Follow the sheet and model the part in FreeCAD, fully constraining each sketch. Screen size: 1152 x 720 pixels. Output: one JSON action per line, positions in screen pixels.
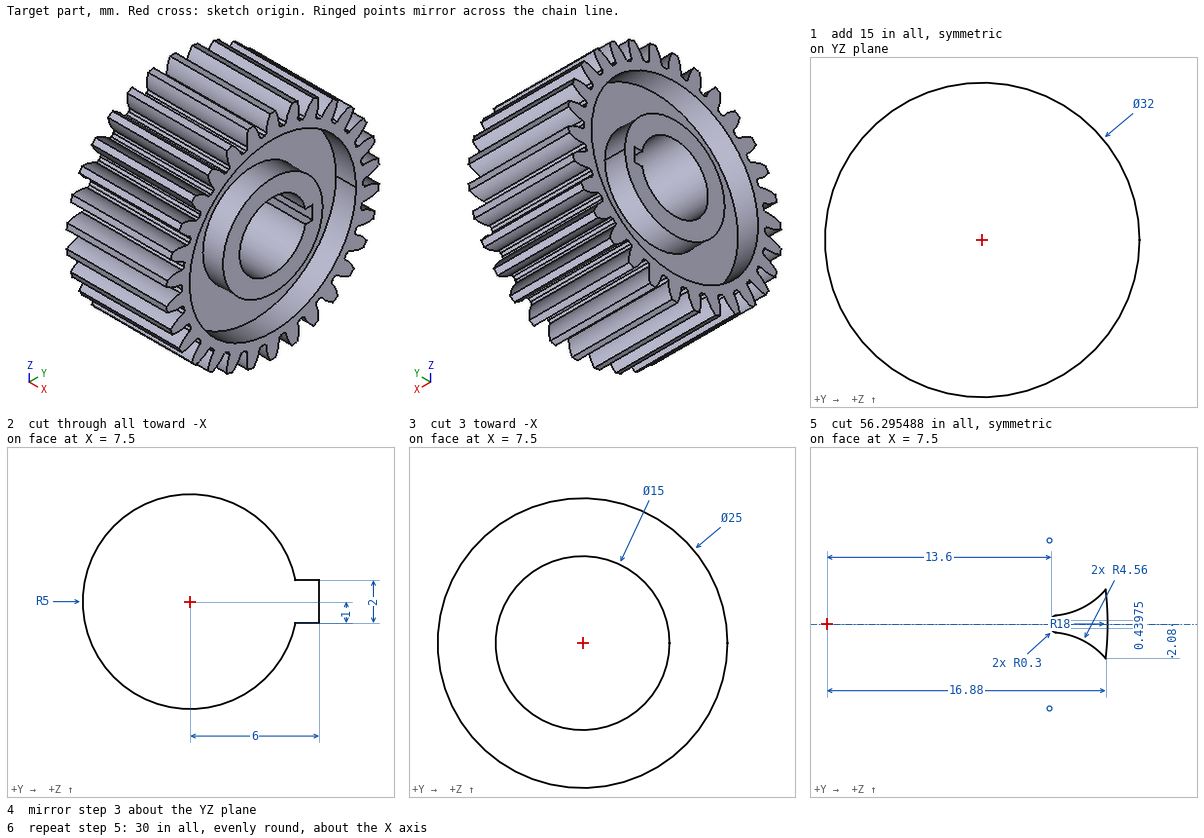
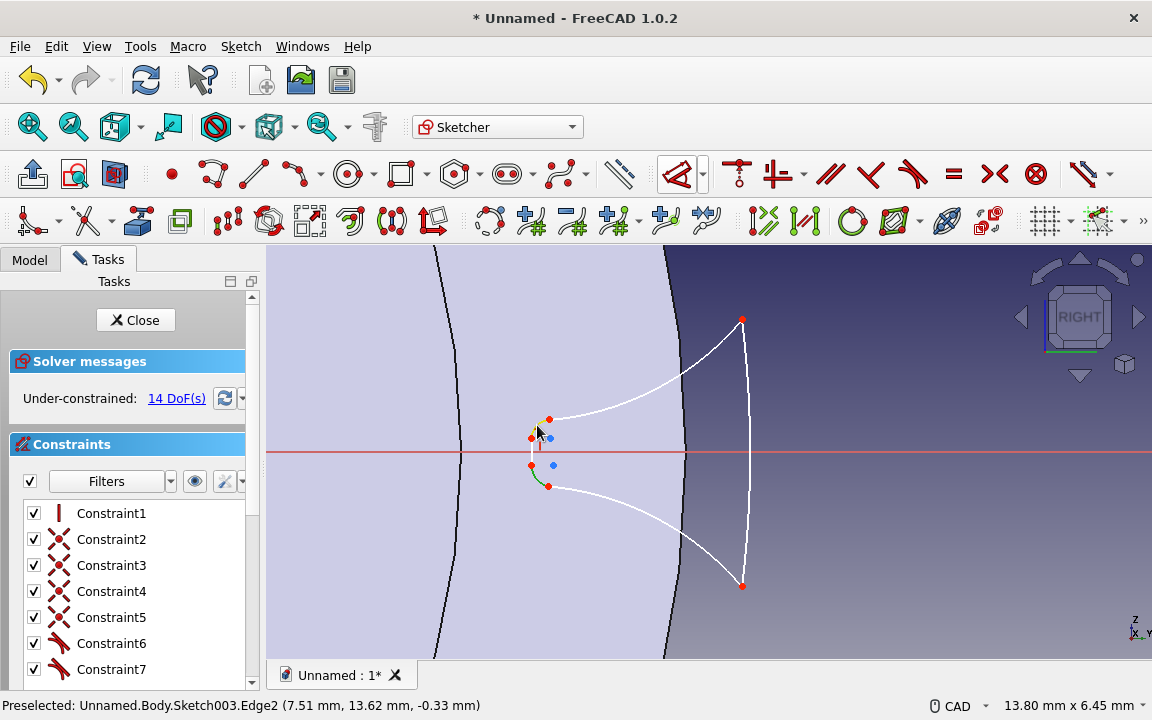
{"action": "left_click", "coordinate": [693, 541]}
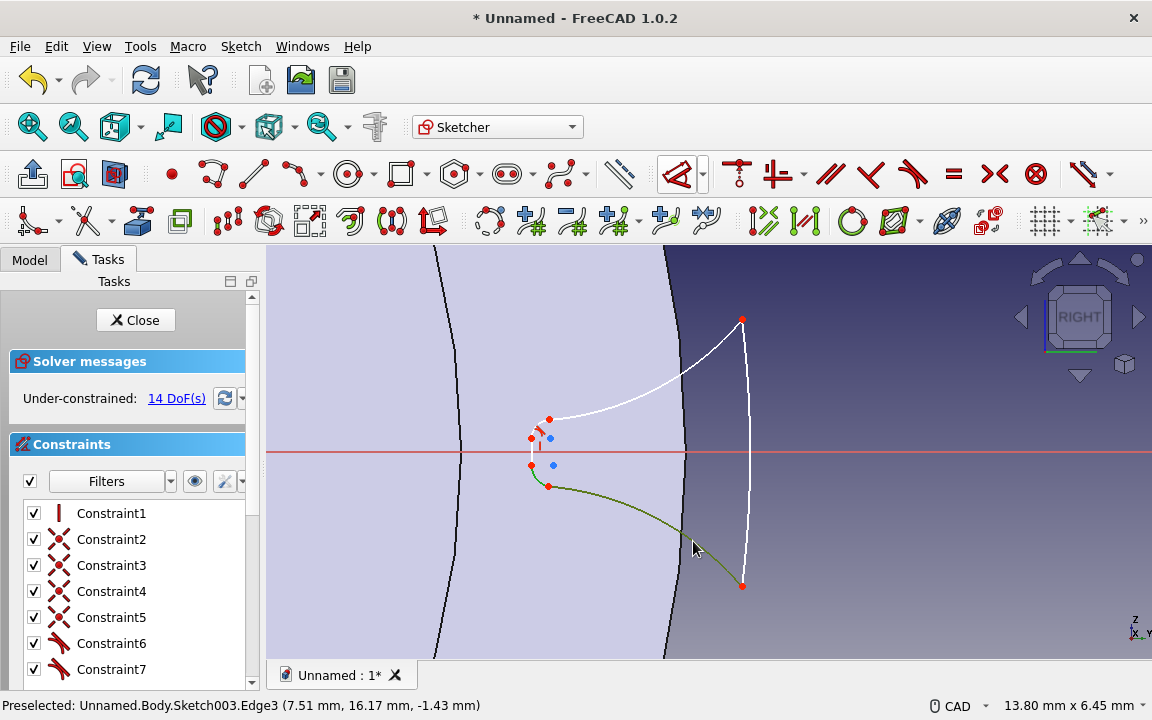
{"action": "left_click", "coordinate": [913, 174]}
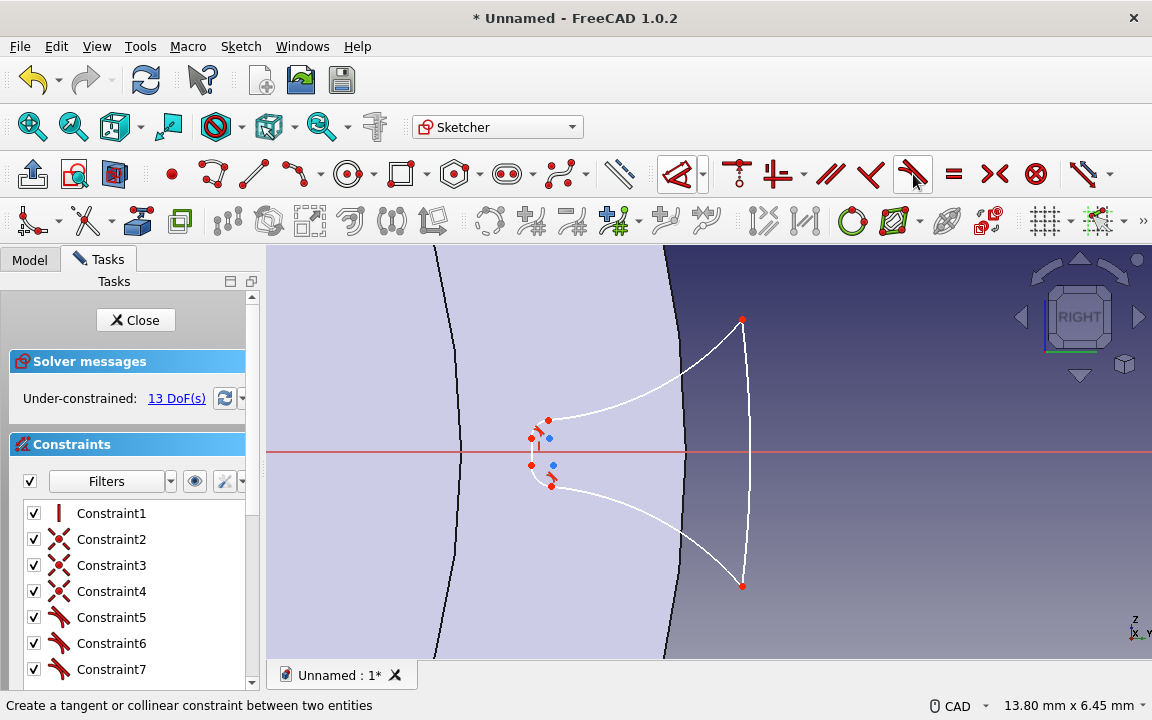
{"action": "left_click", "coordinate": [614, 407]}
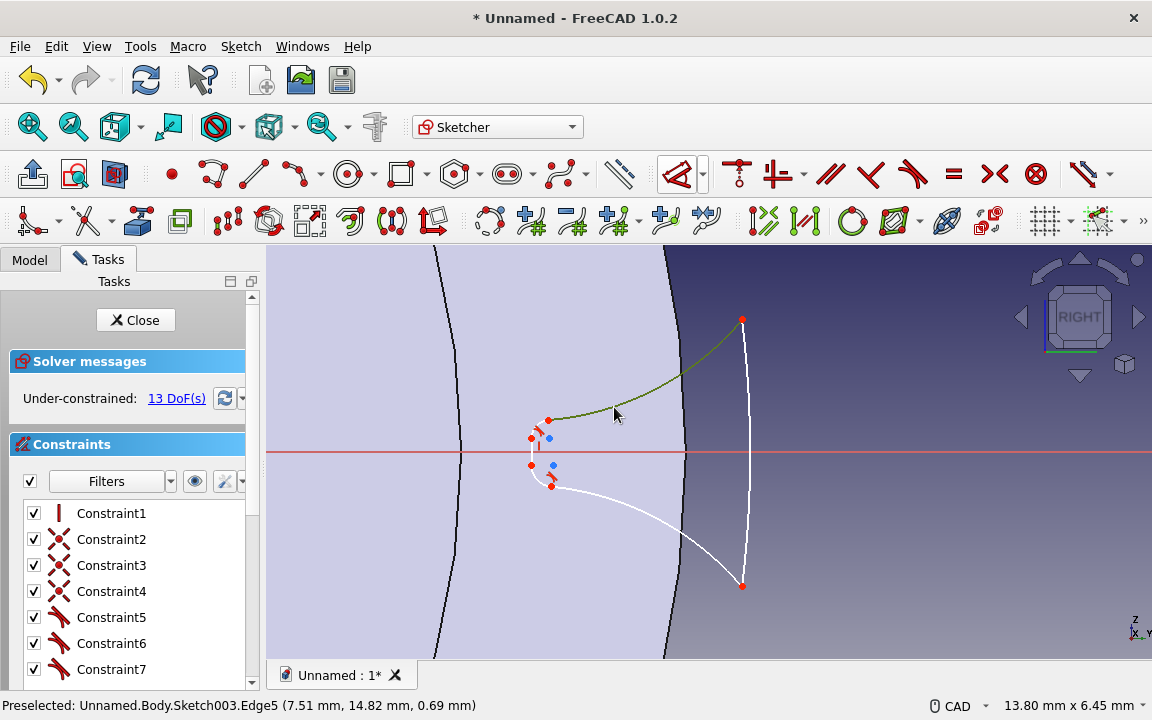
{"action": "left_click", "coordinate": [541, 422]}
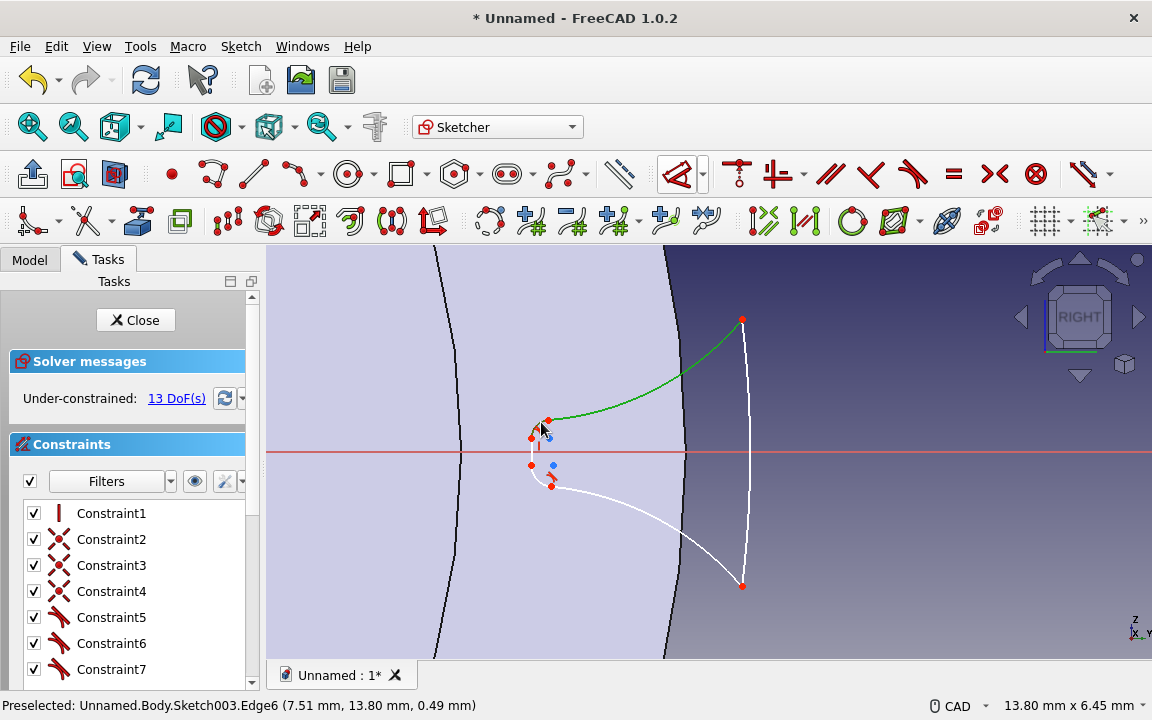
{"action": "key", "text": "t"}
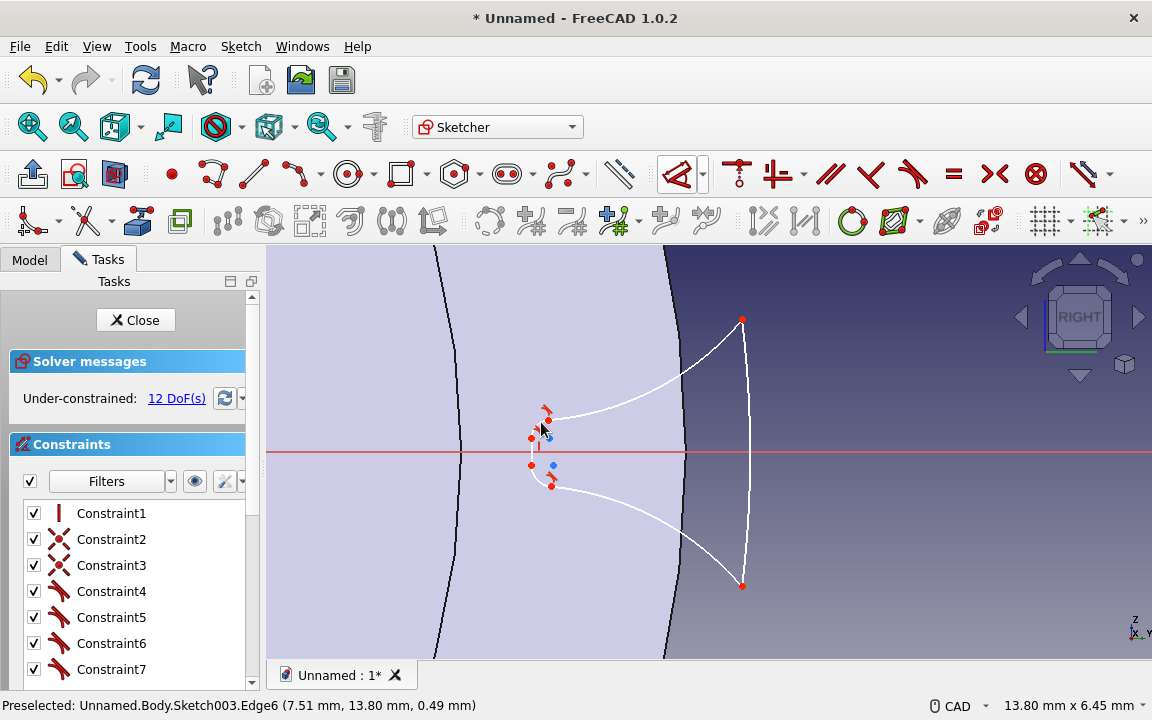
{"action": "left_click", "coordinate": [694, 542]}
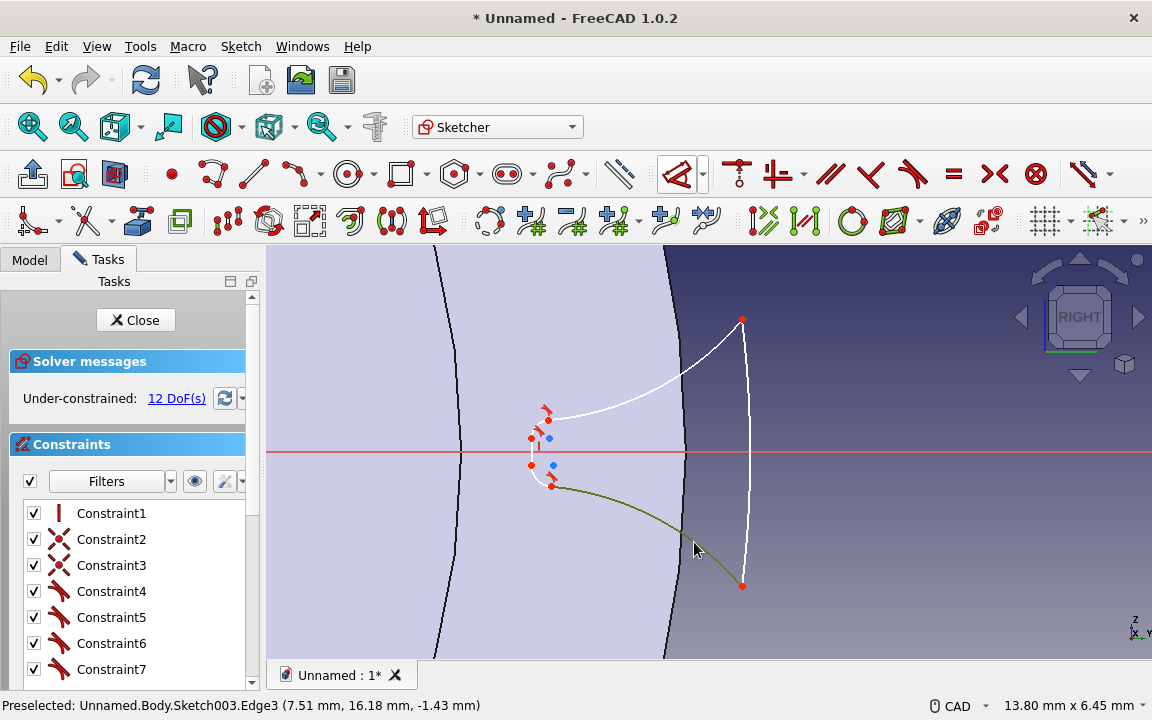
{"action": "left_click", "coordinate": [614, 407]}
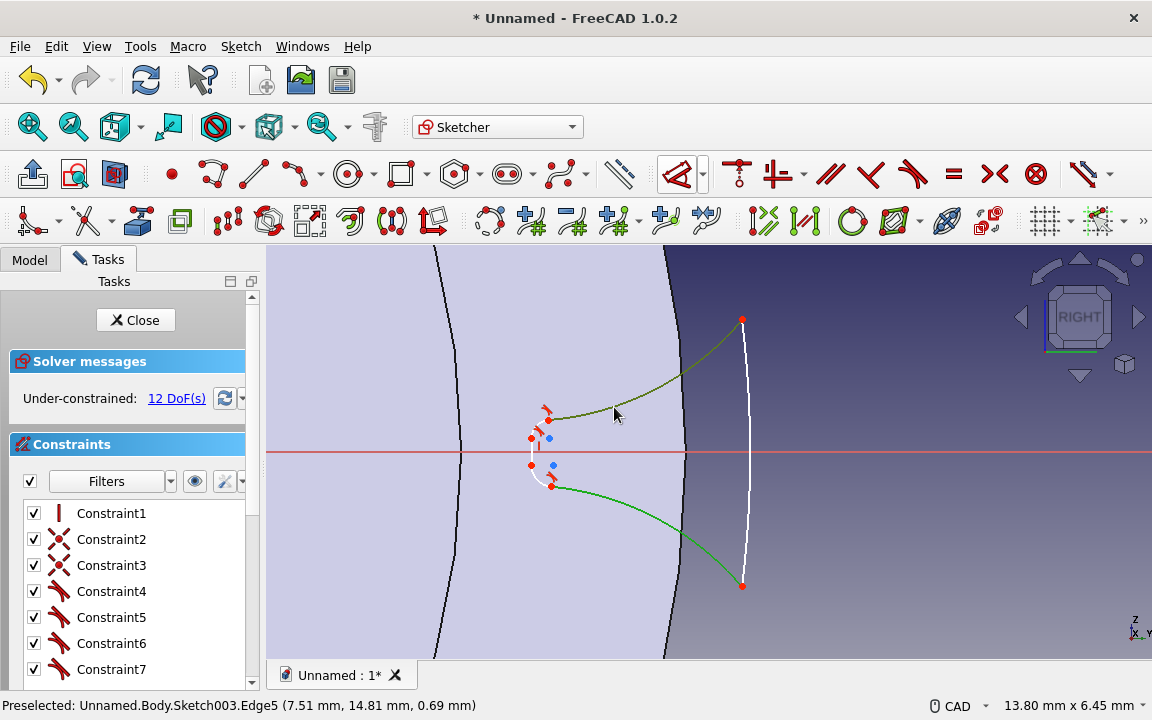
{"action": "key", "text": "e"}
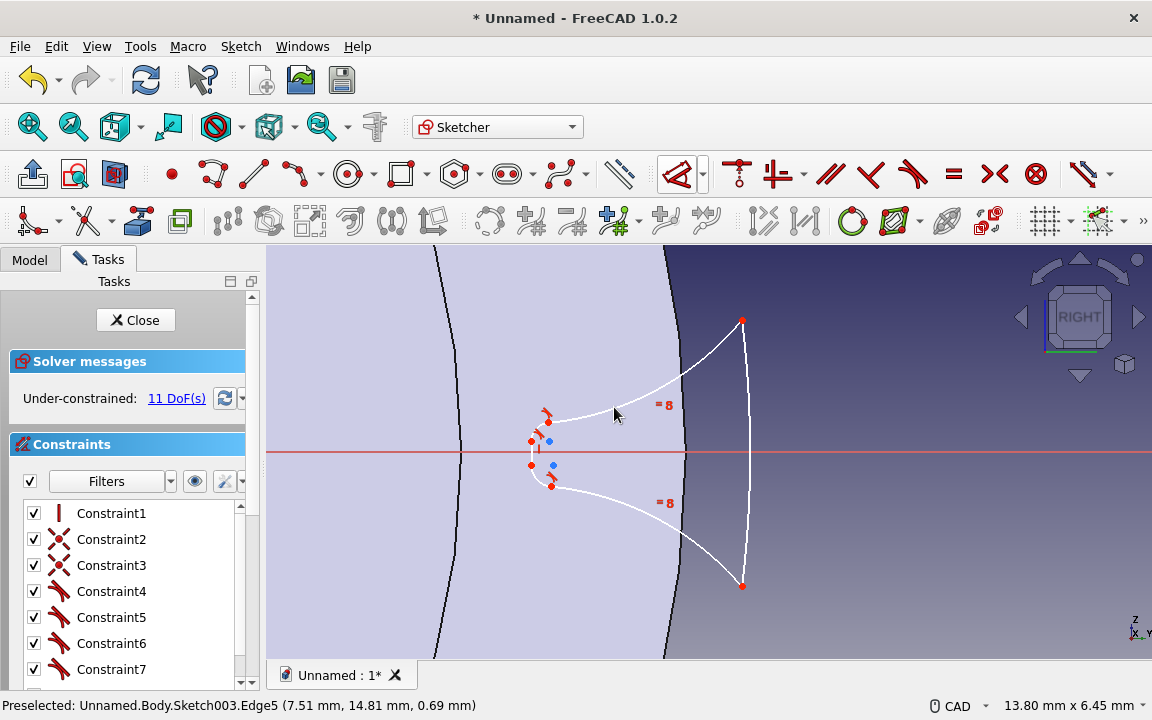
{"action": "scroll", "coordinate": [534, 474], "scroll_direction": "up", "scroll_amount": 2}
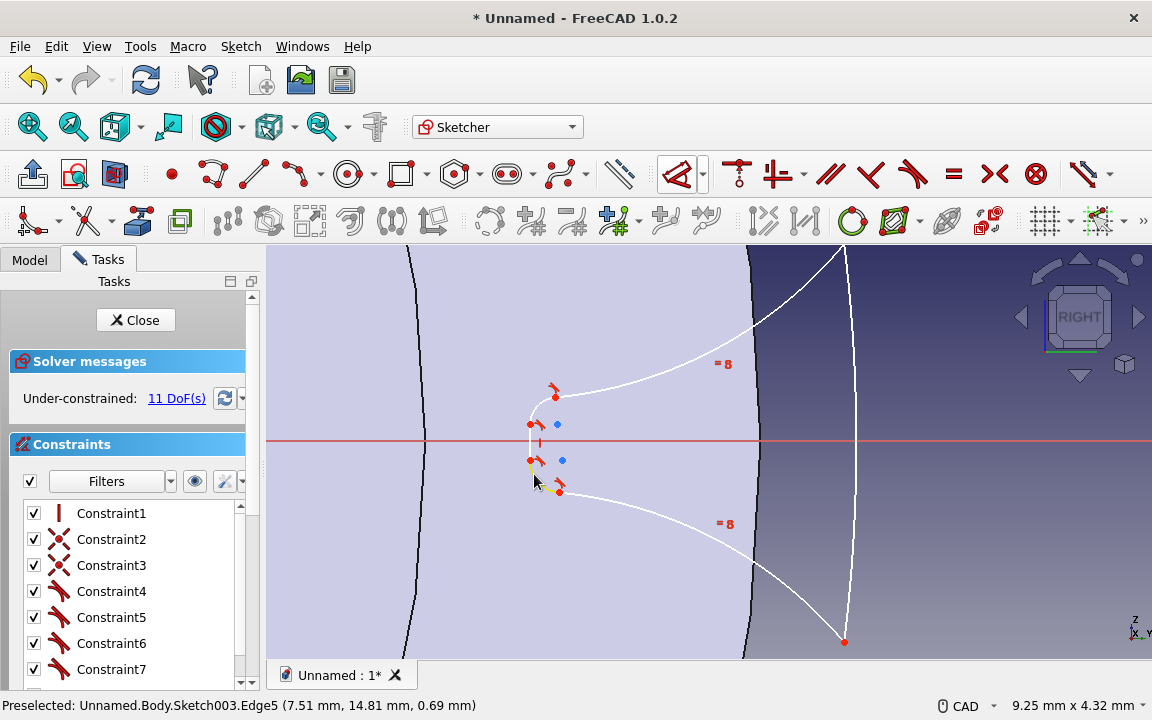
{"action": "left_click", "coordinate": [533, 474]}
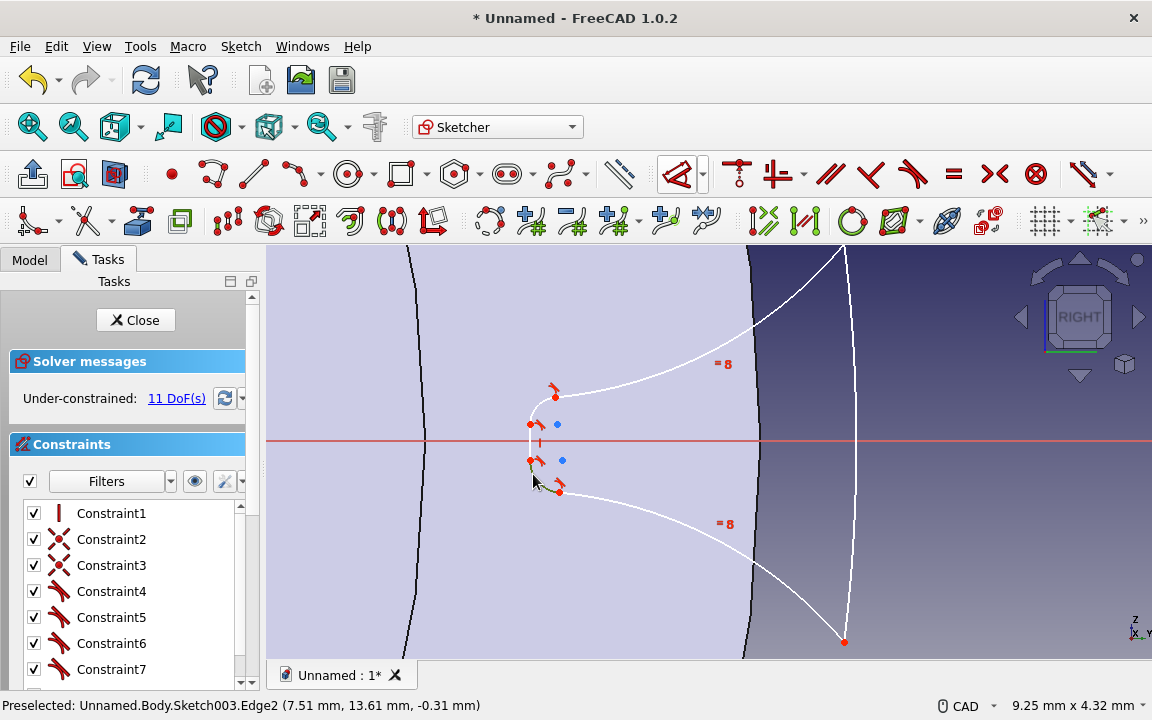
{"action": "left_click", "coordinate": [544, 401]}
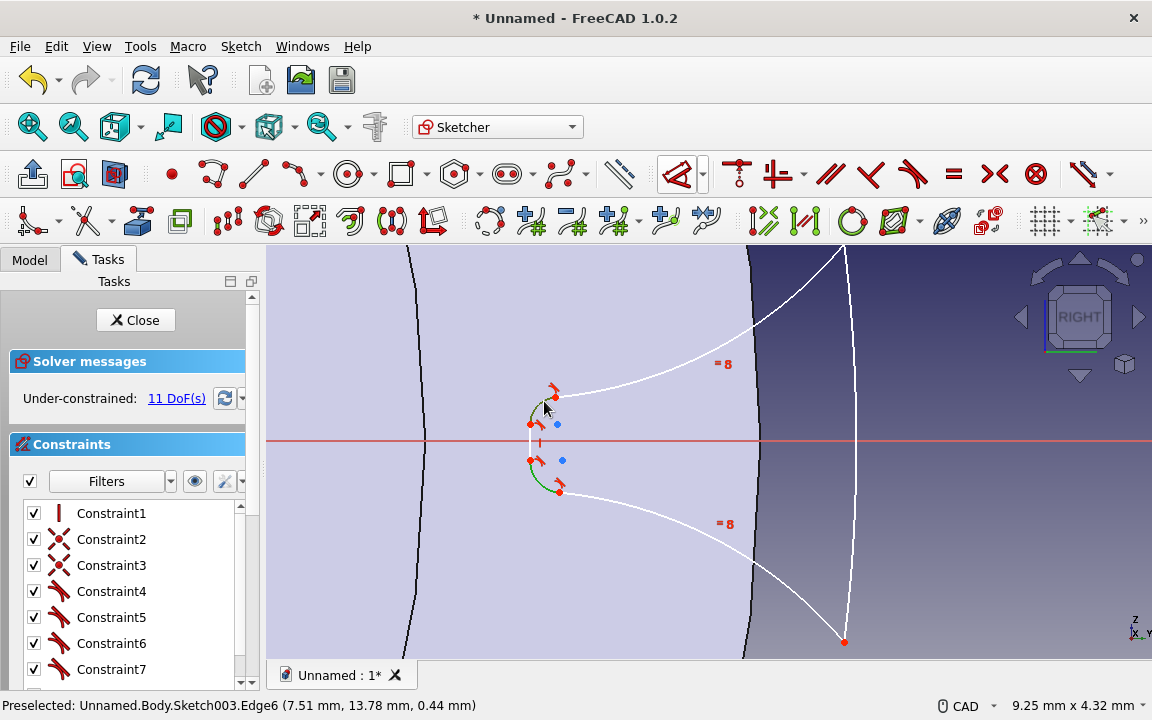
{"action": "key", "text": "e"}